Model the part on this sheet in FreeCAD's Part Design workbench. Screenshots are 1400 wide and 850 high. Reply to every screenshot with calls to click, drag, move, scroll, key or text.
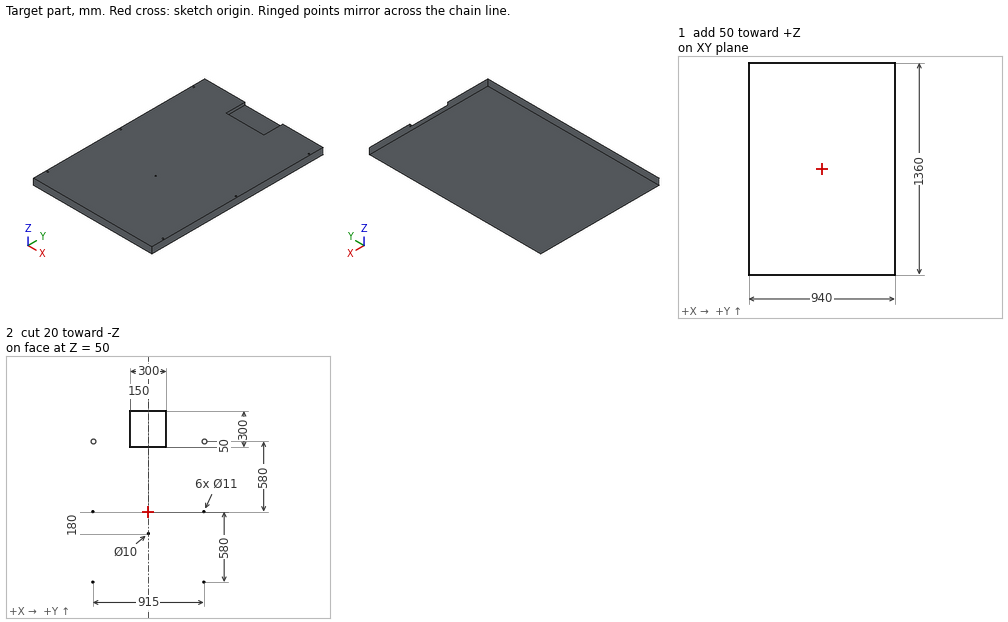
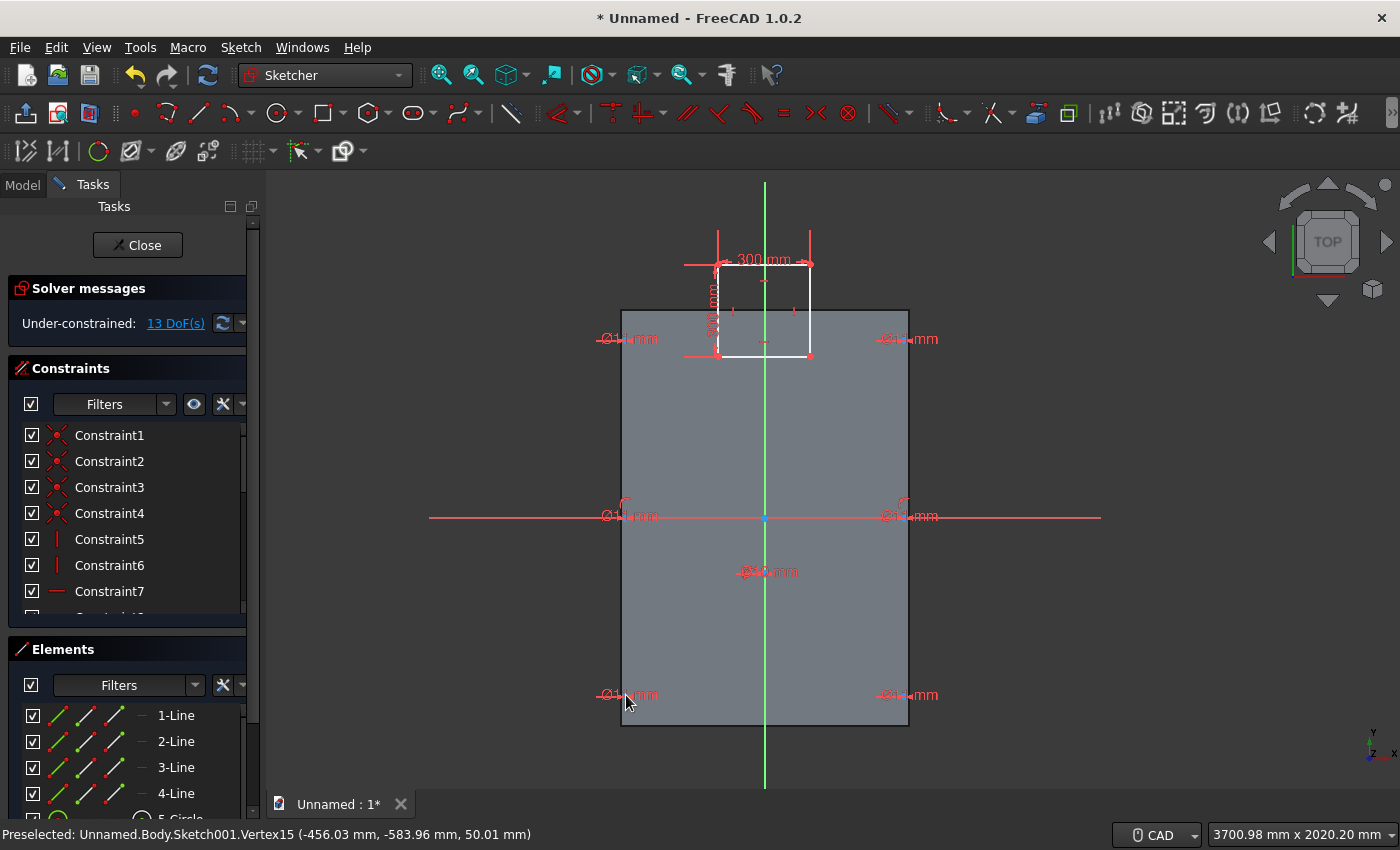
click(905, 697)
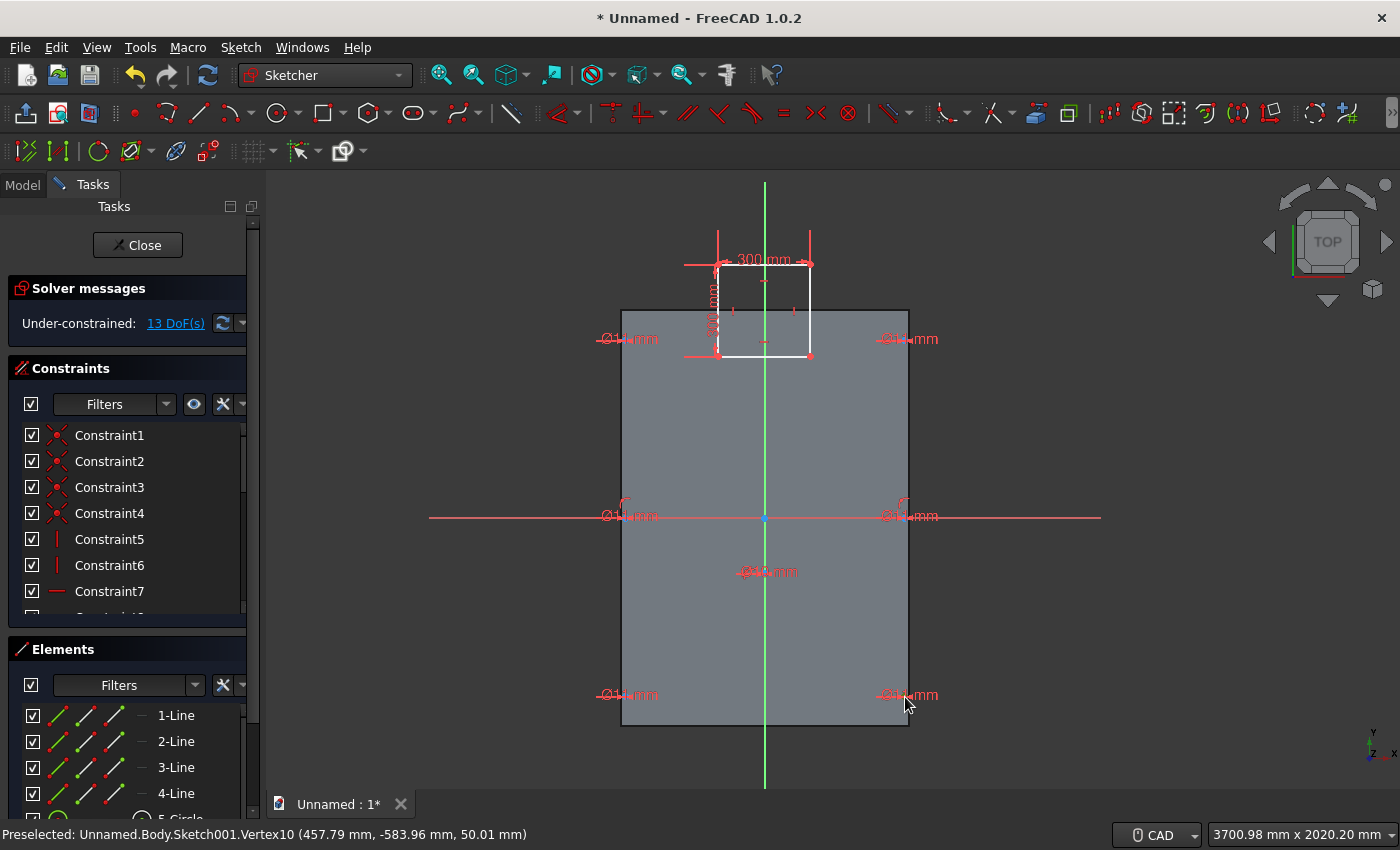
click(905, 518)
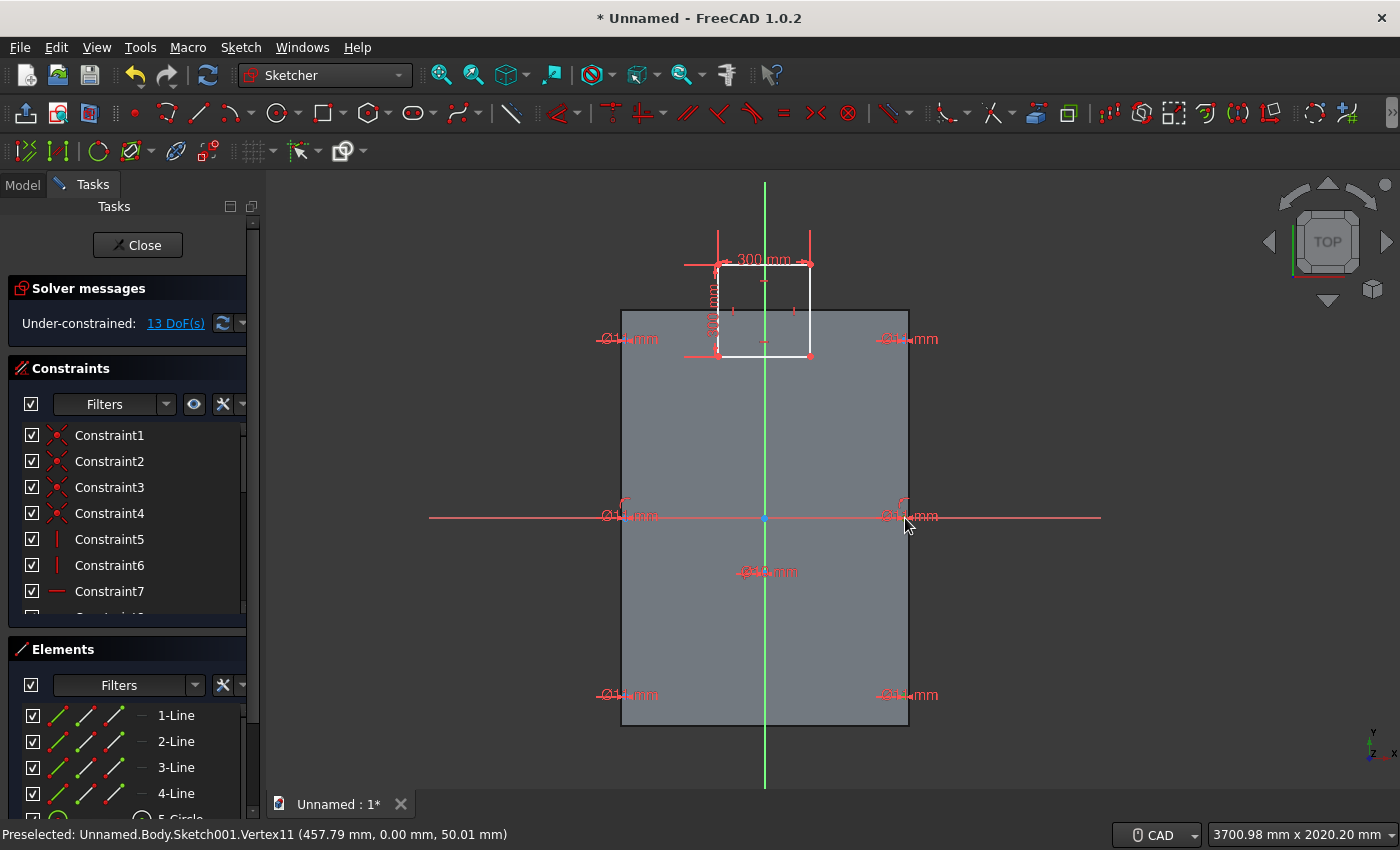
key(v)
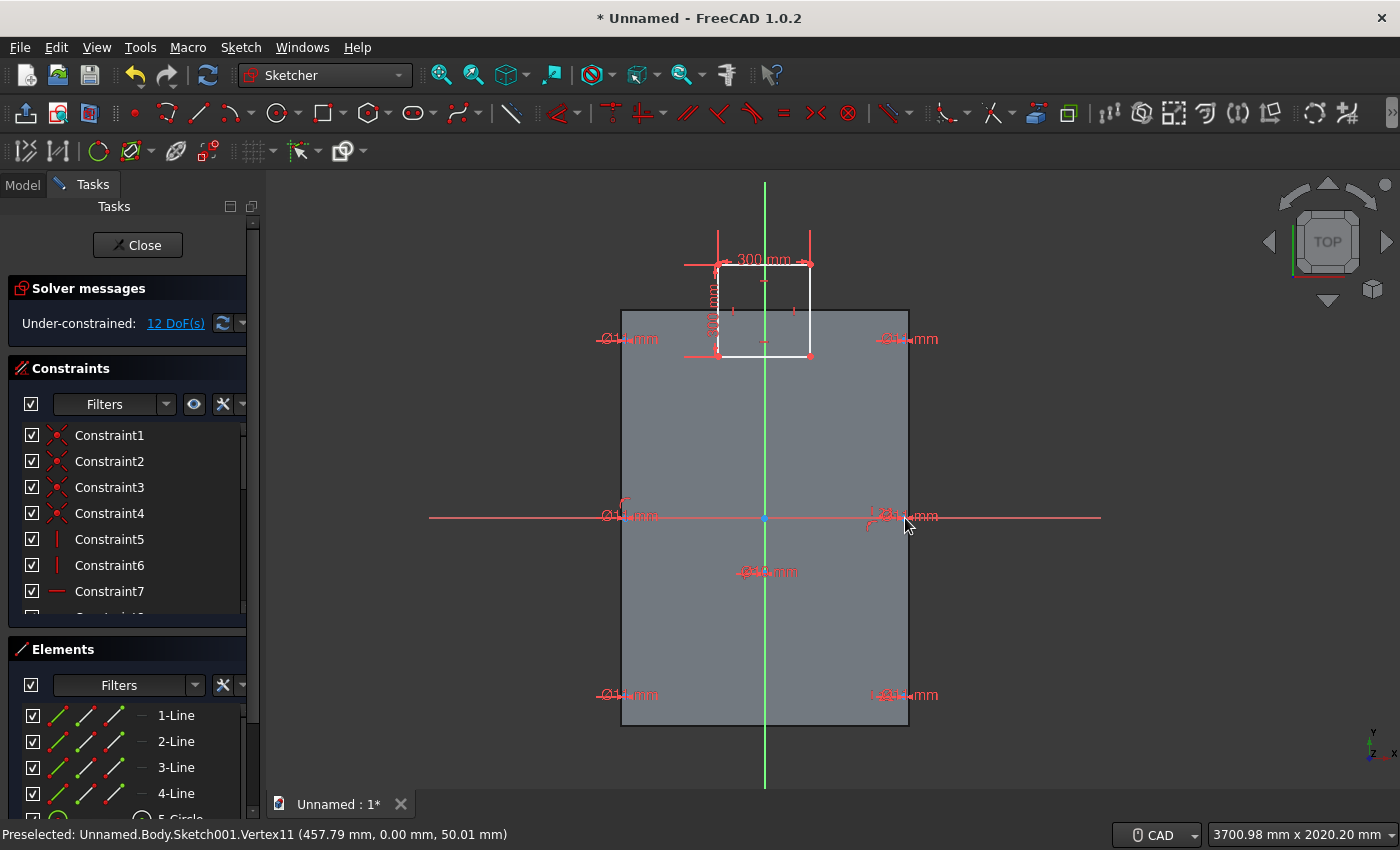
click(905, 518)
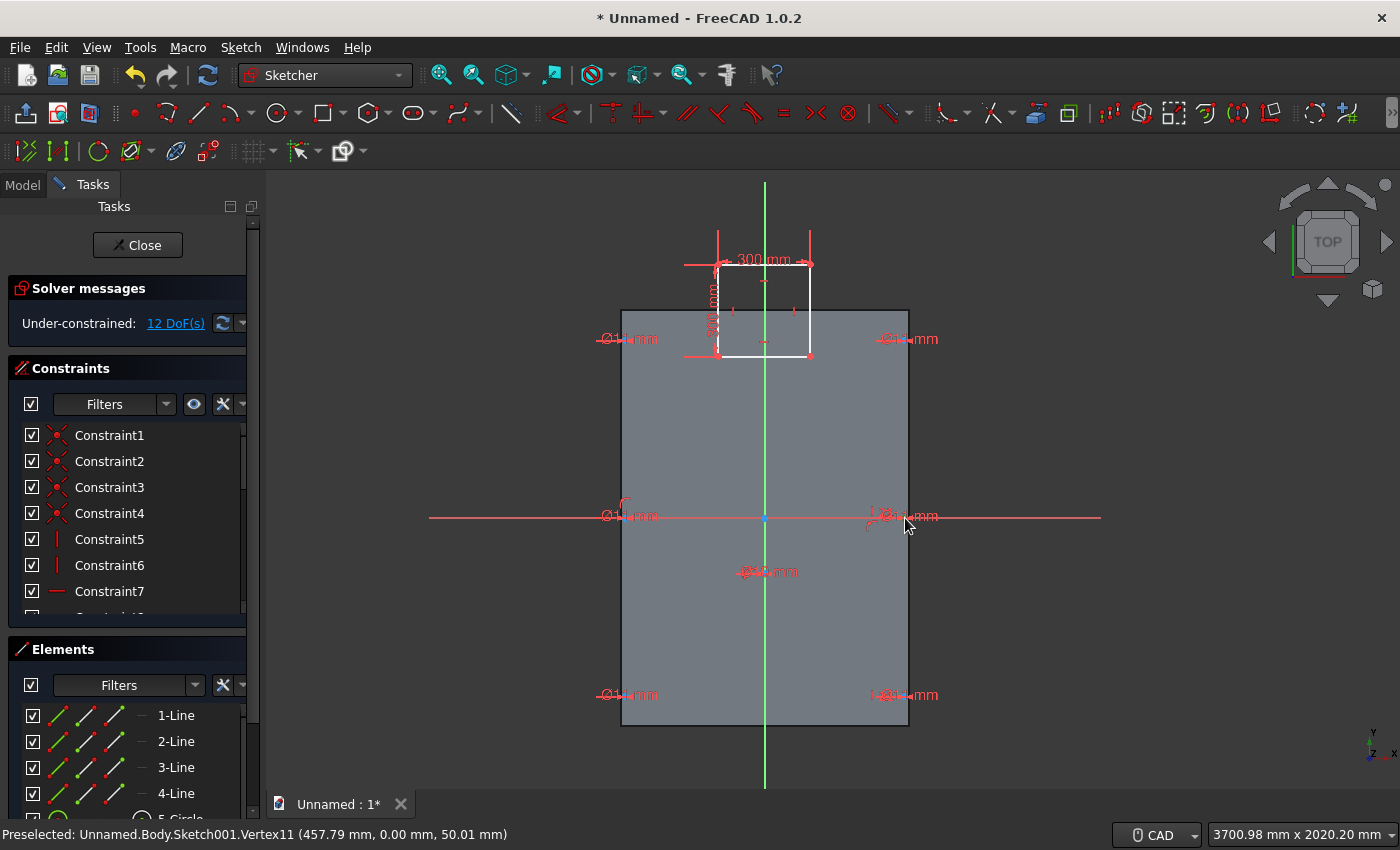
click(905, 341)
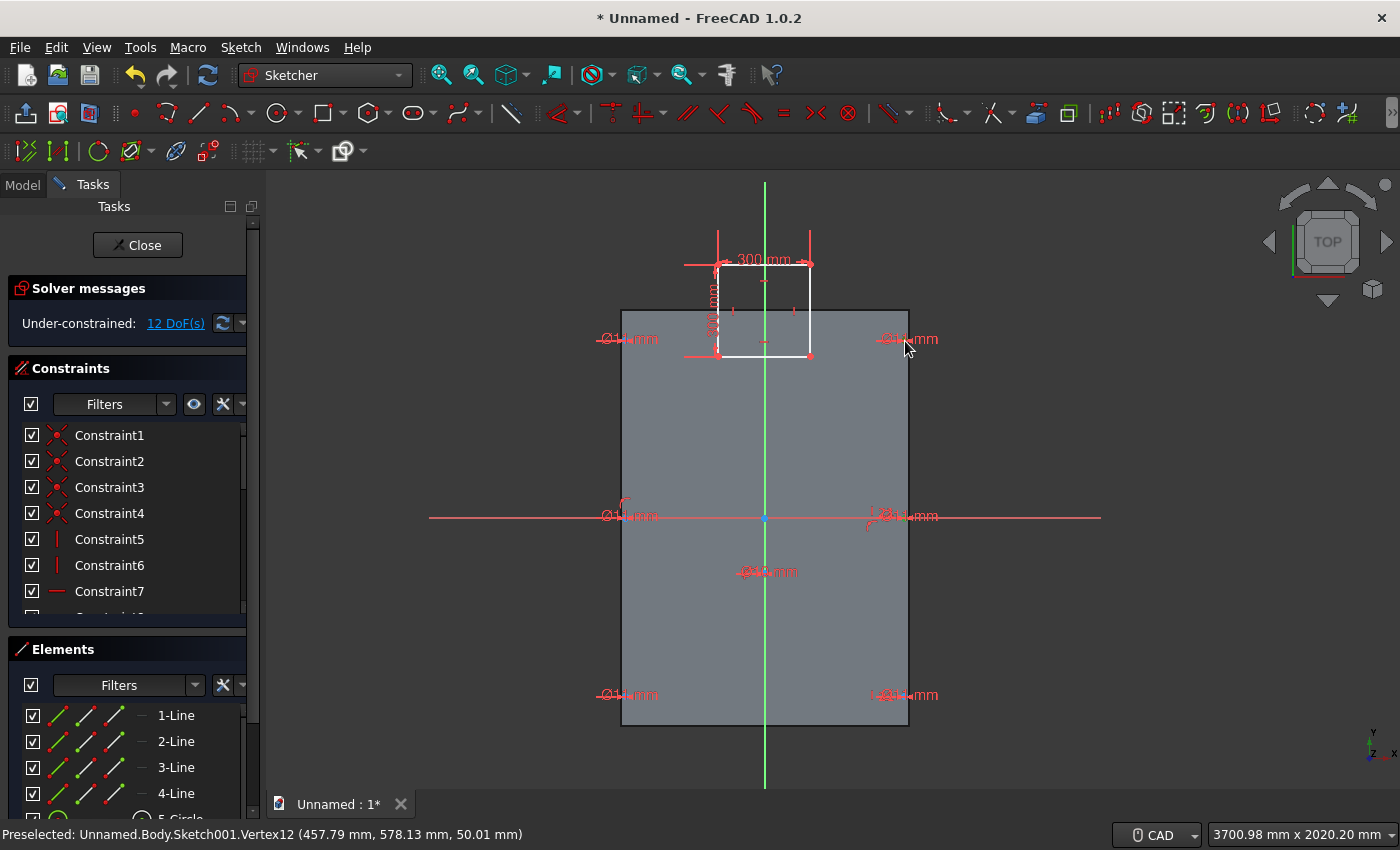
key(v)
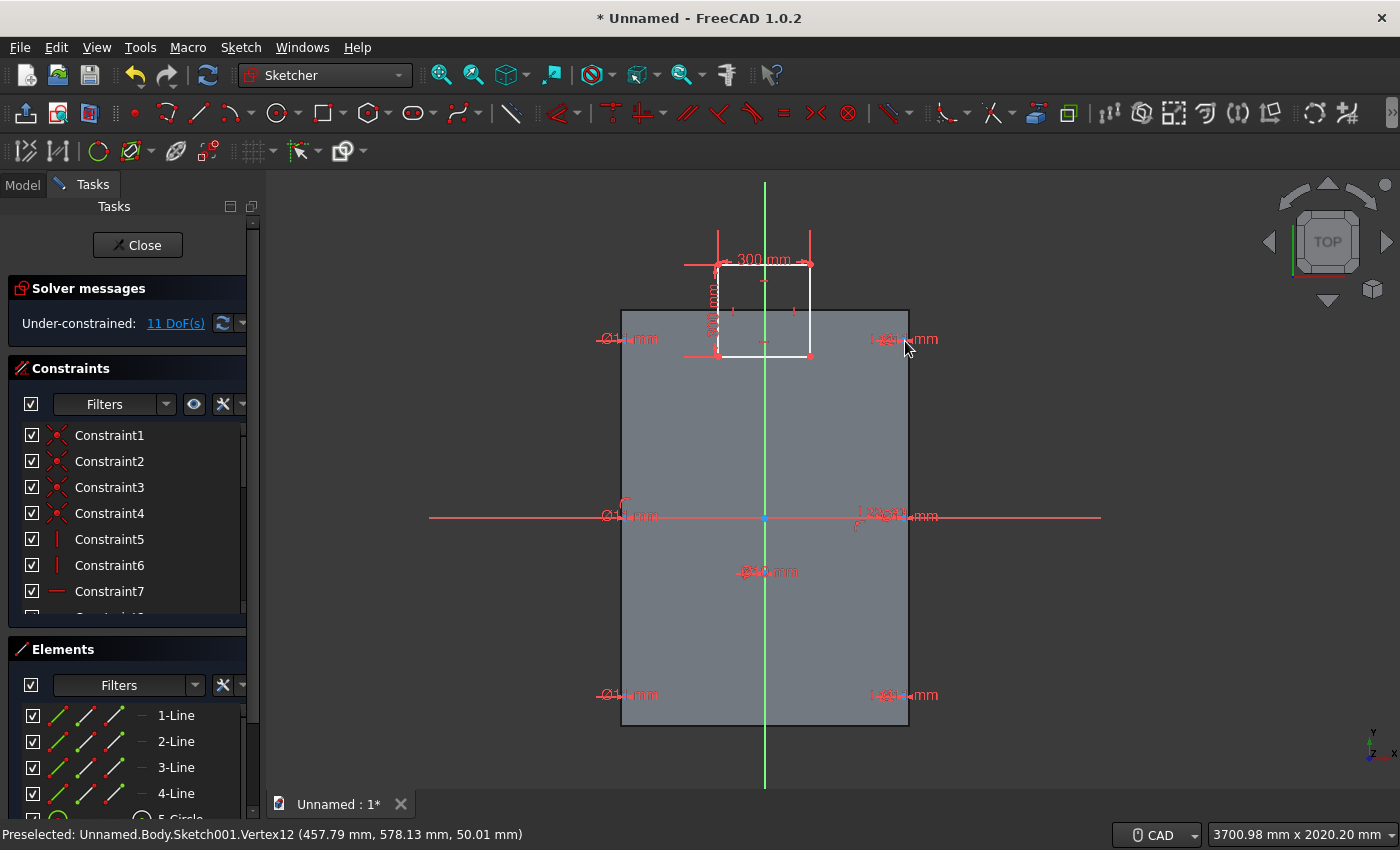
click(625, 341)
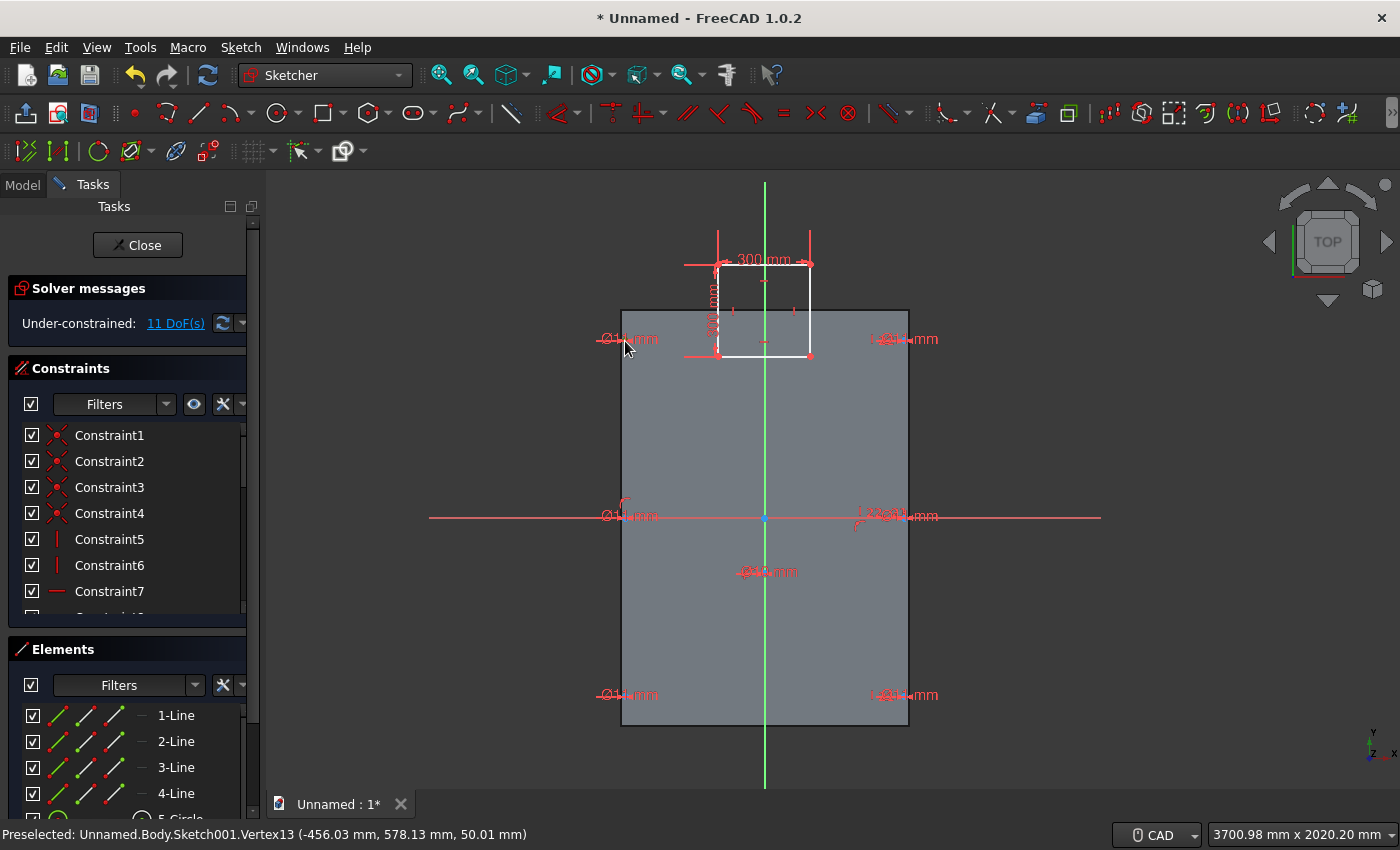
click(625, 518)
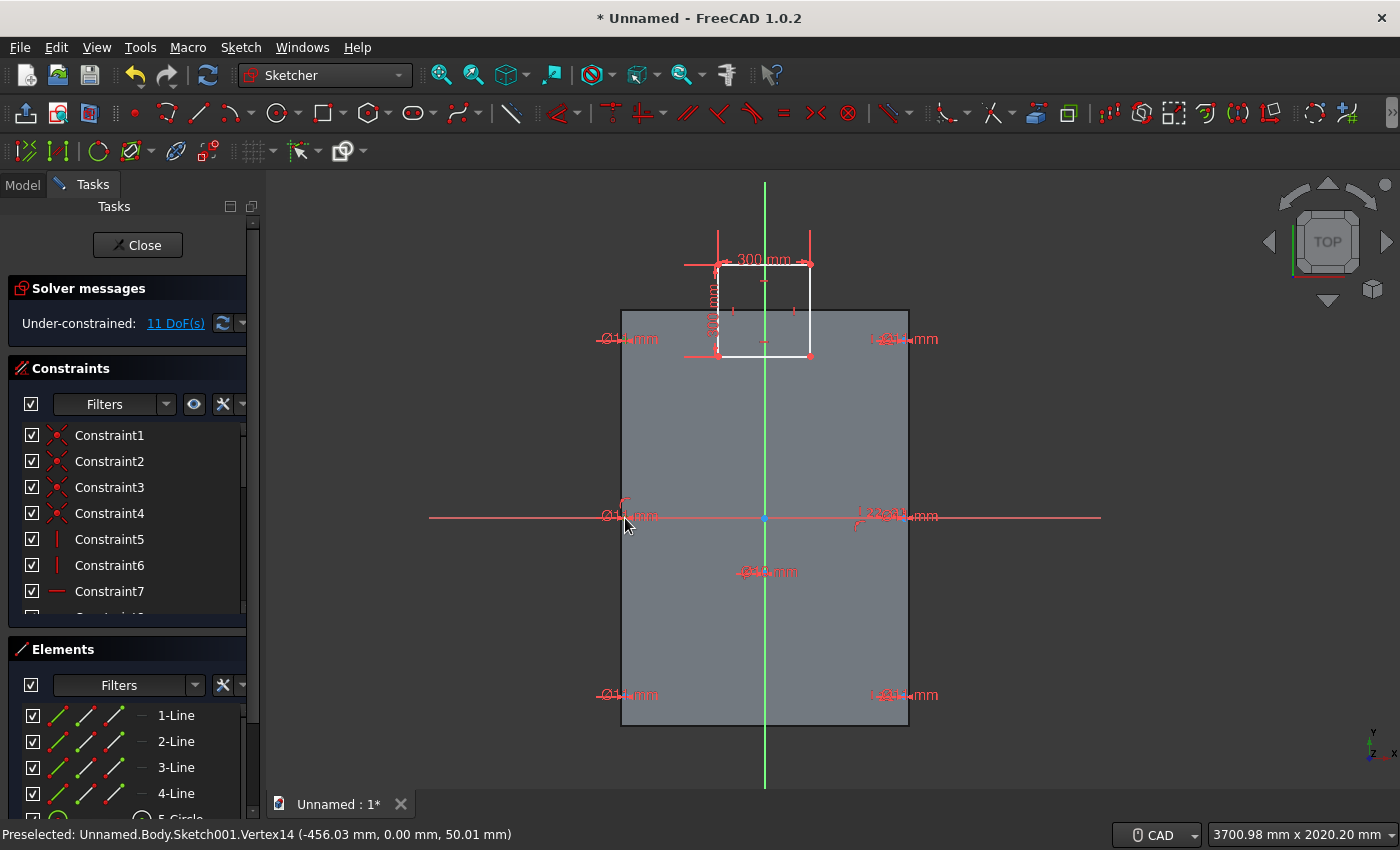
key(v)